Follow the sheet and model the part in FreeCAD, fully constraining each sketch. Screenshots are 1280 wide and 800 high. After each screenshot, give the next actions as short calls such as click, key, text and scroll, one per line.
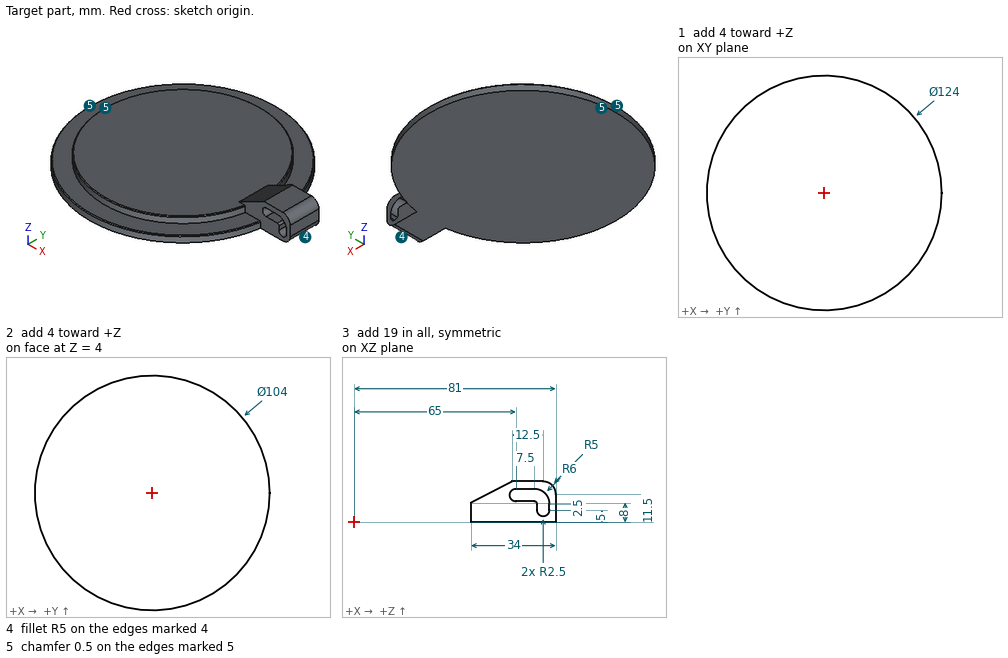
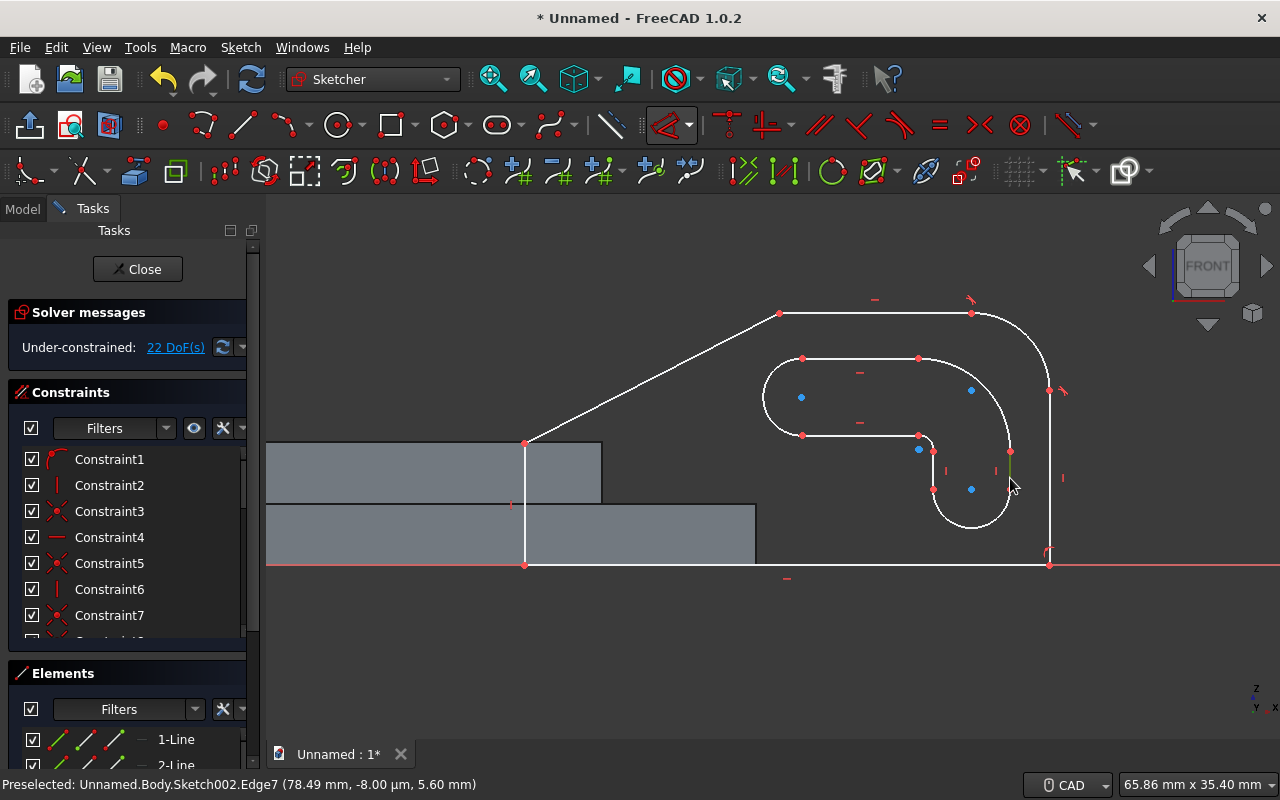
click(1001, 409)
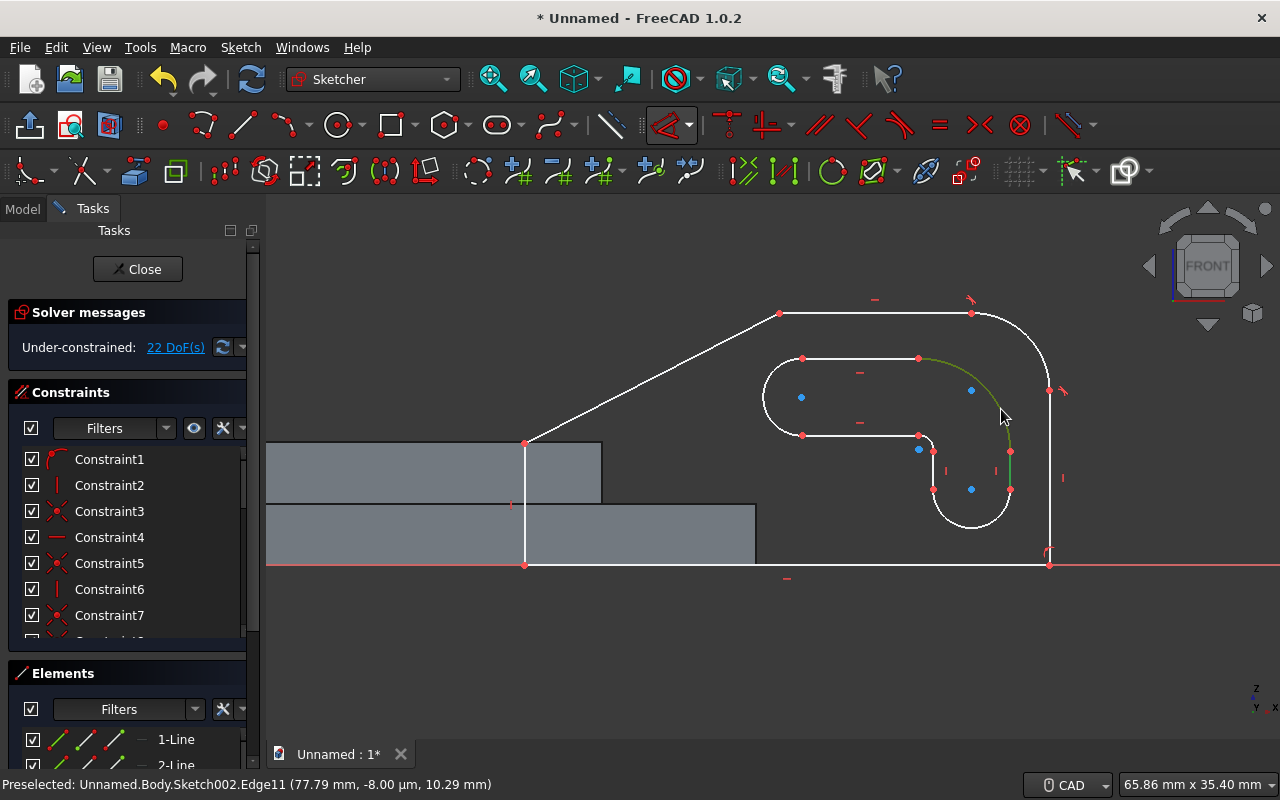
click(900, 126)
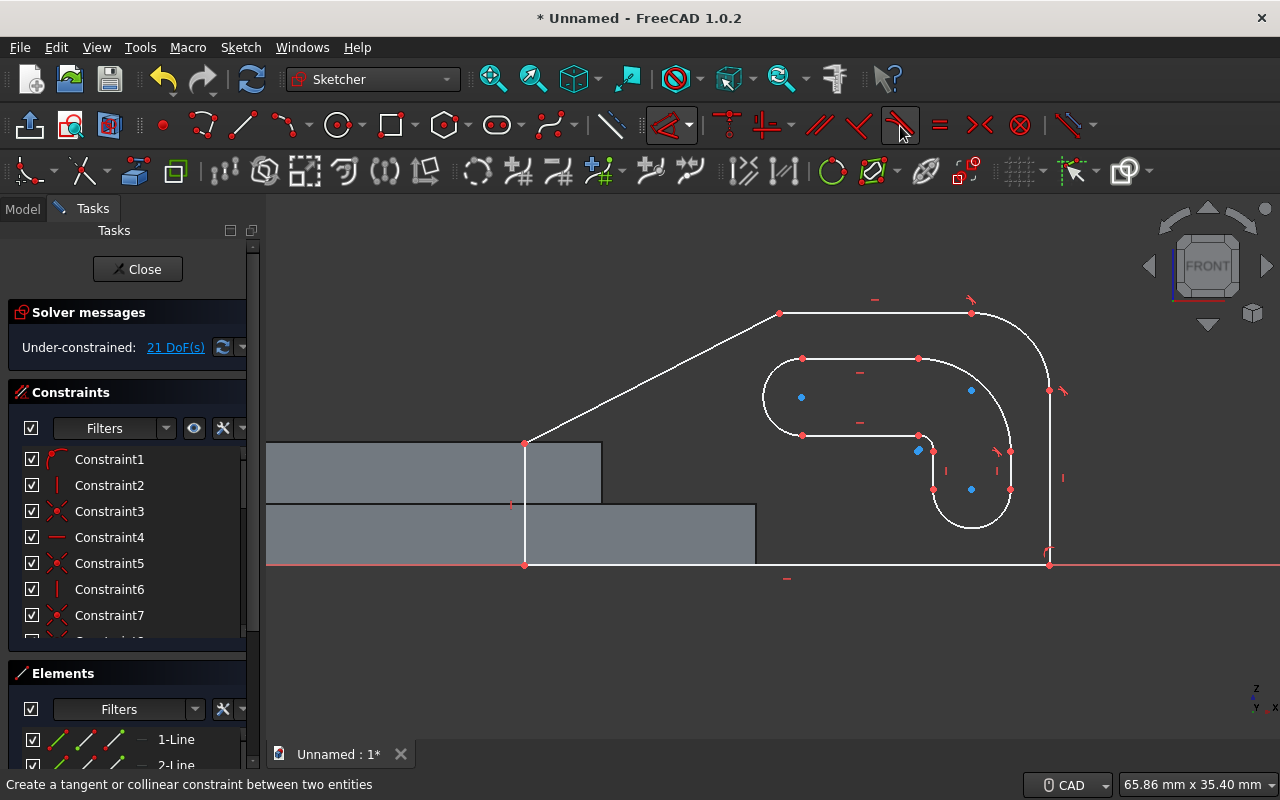
click(1011, 478)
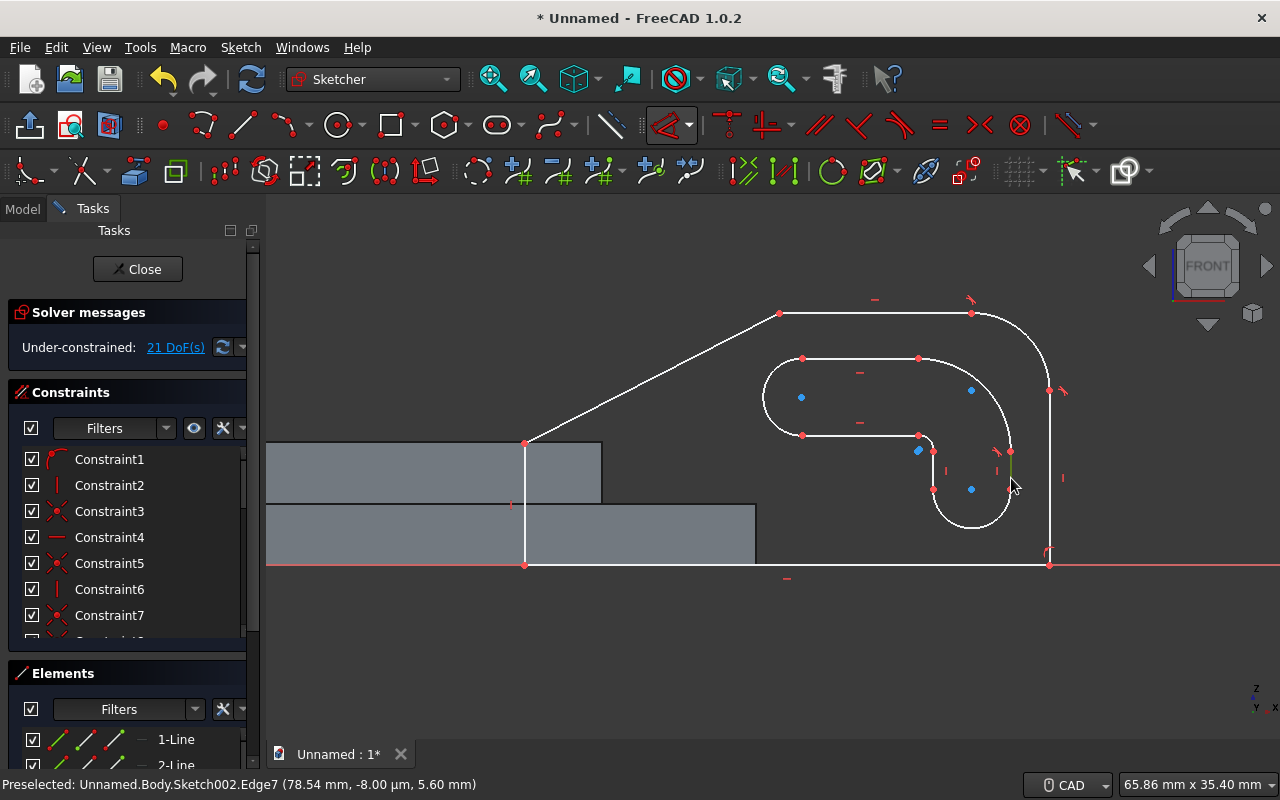
click(949, 521)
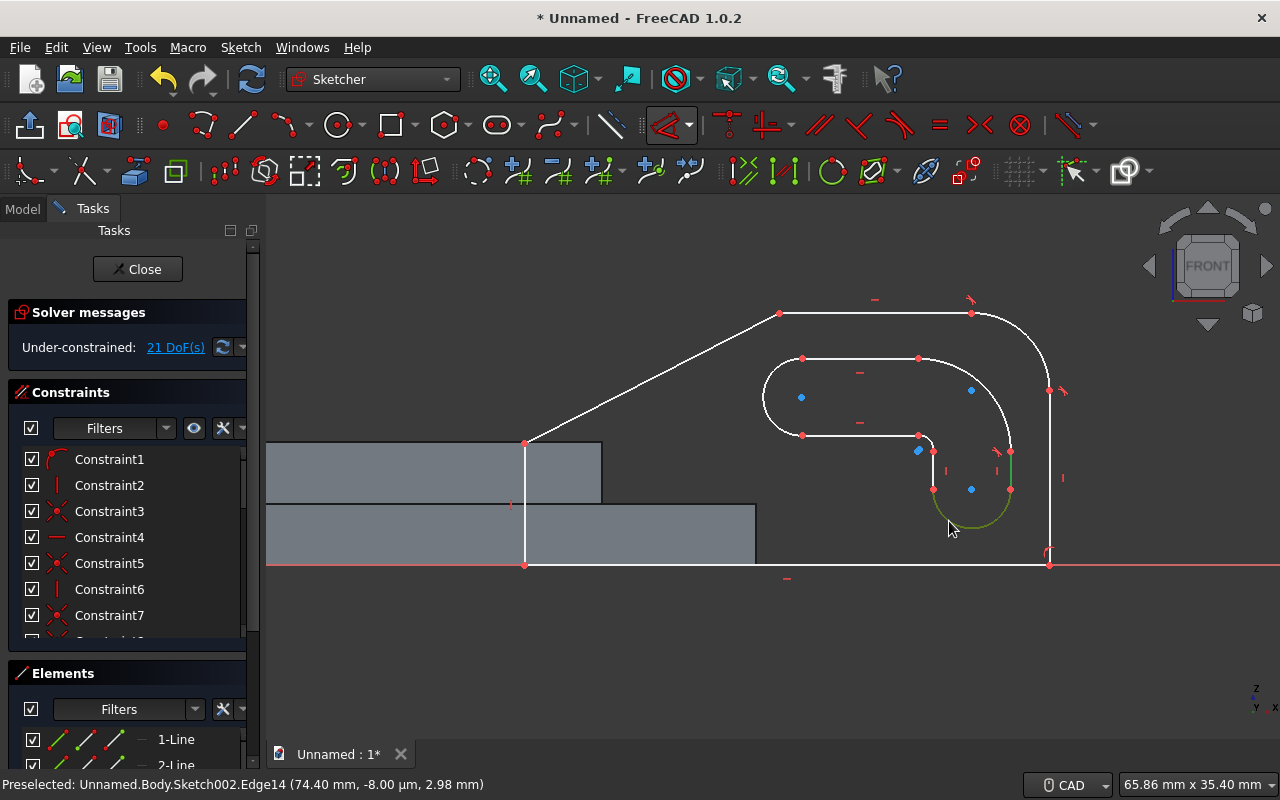
click(900, 126)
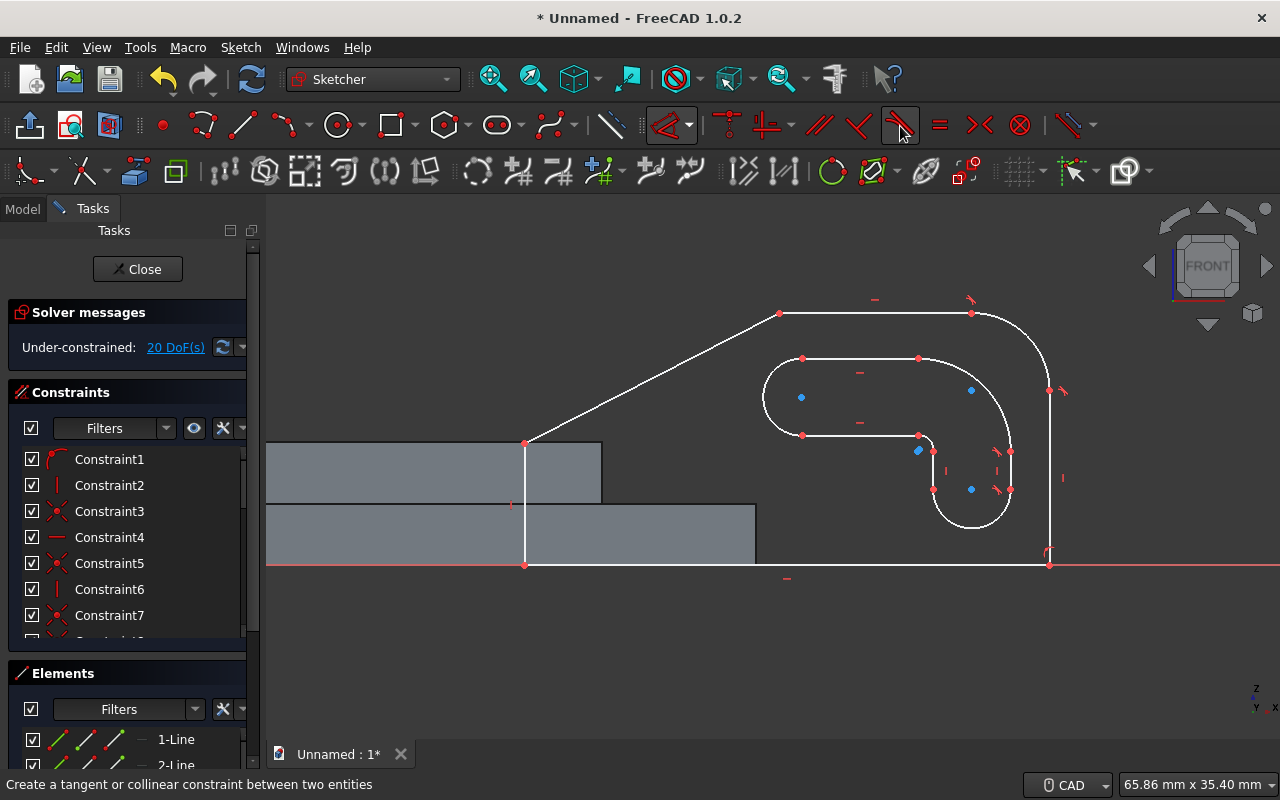
click(884, 359)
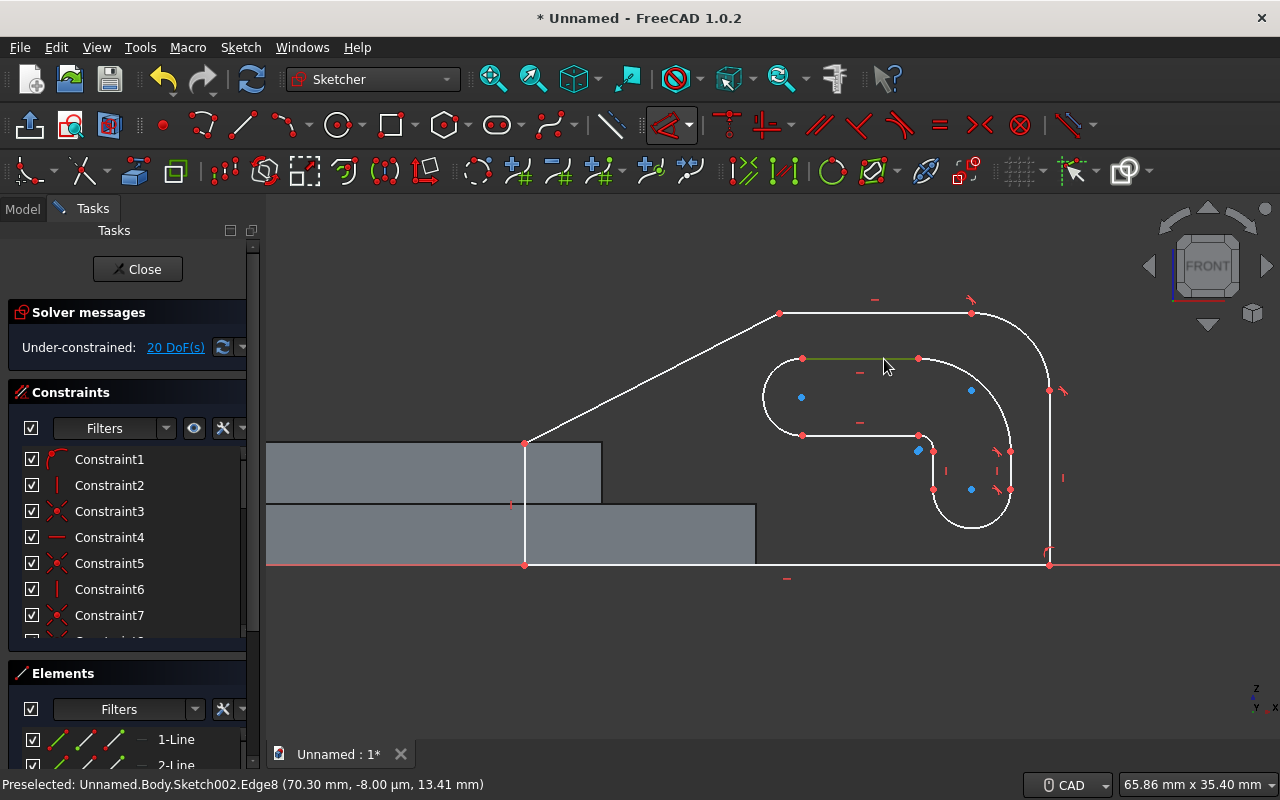
click(1001, 410)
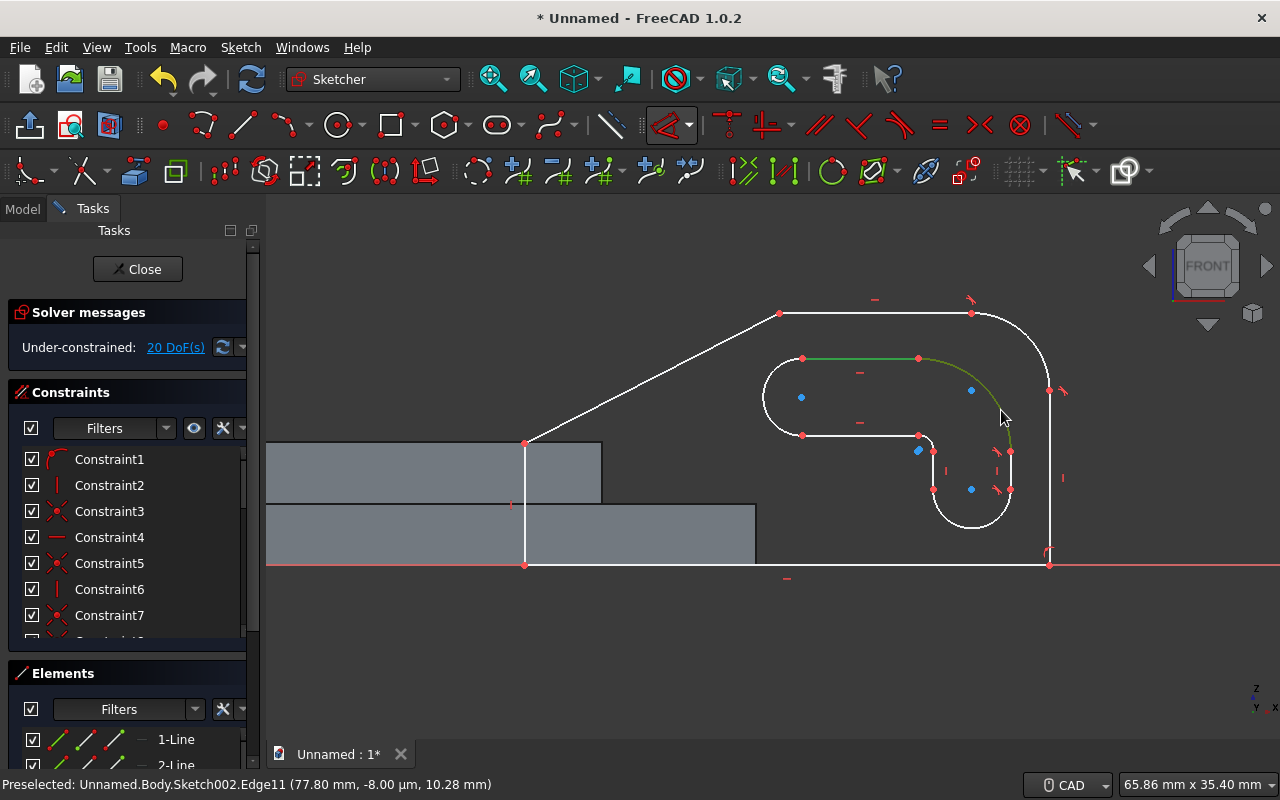
click(900, 126)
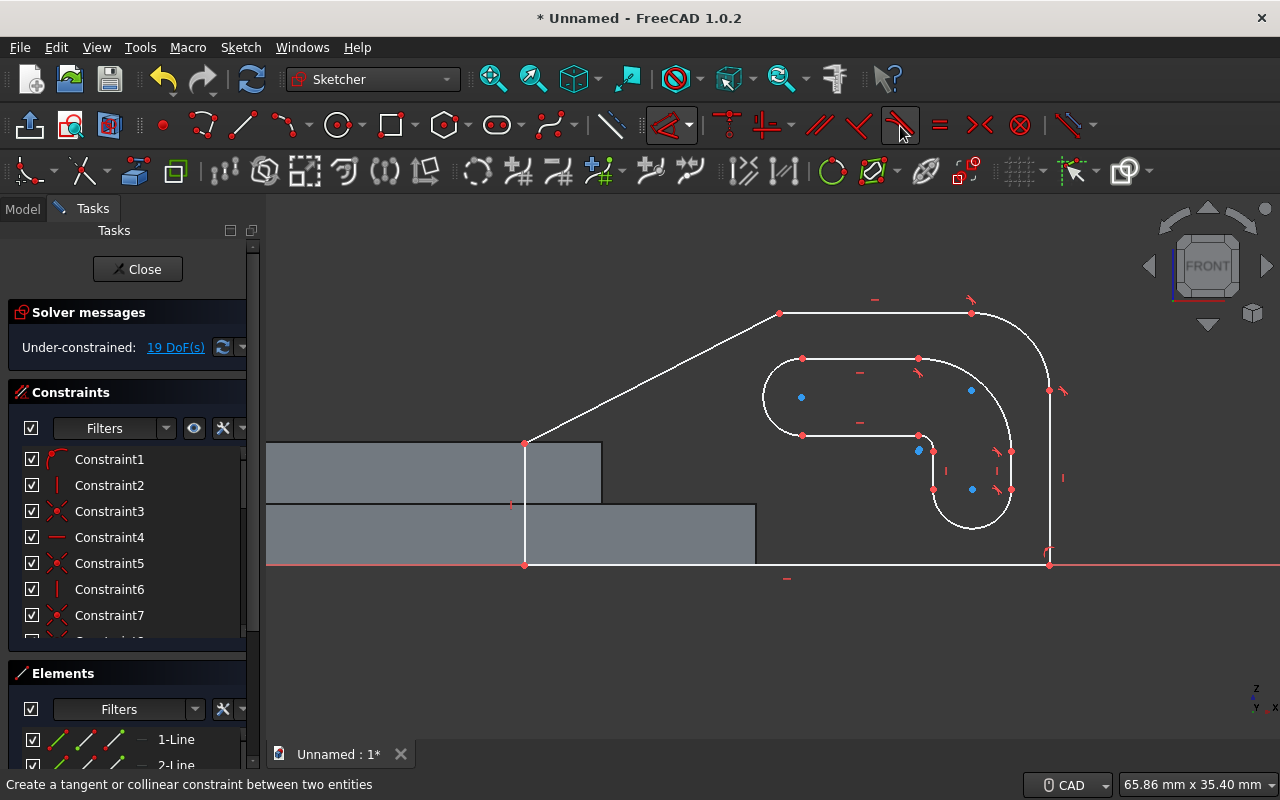
click(884, 359)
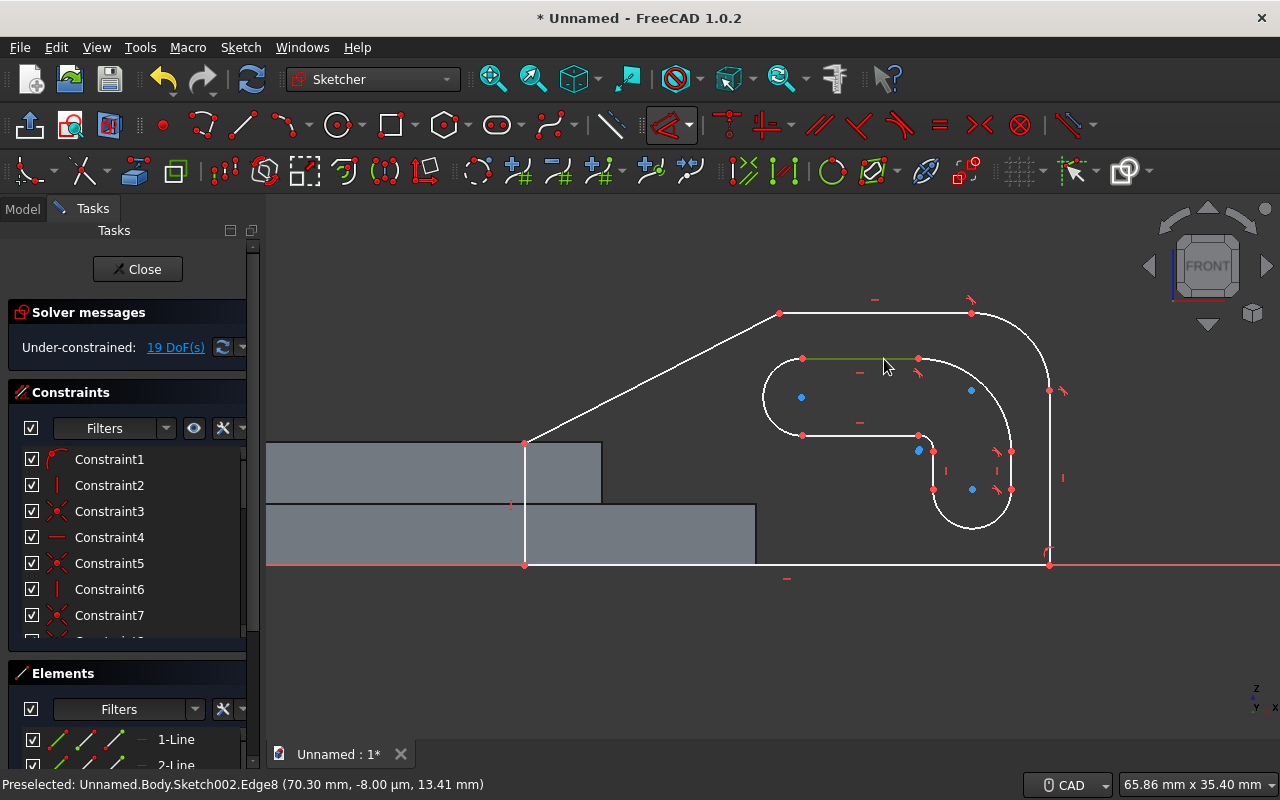
click(771, 374)